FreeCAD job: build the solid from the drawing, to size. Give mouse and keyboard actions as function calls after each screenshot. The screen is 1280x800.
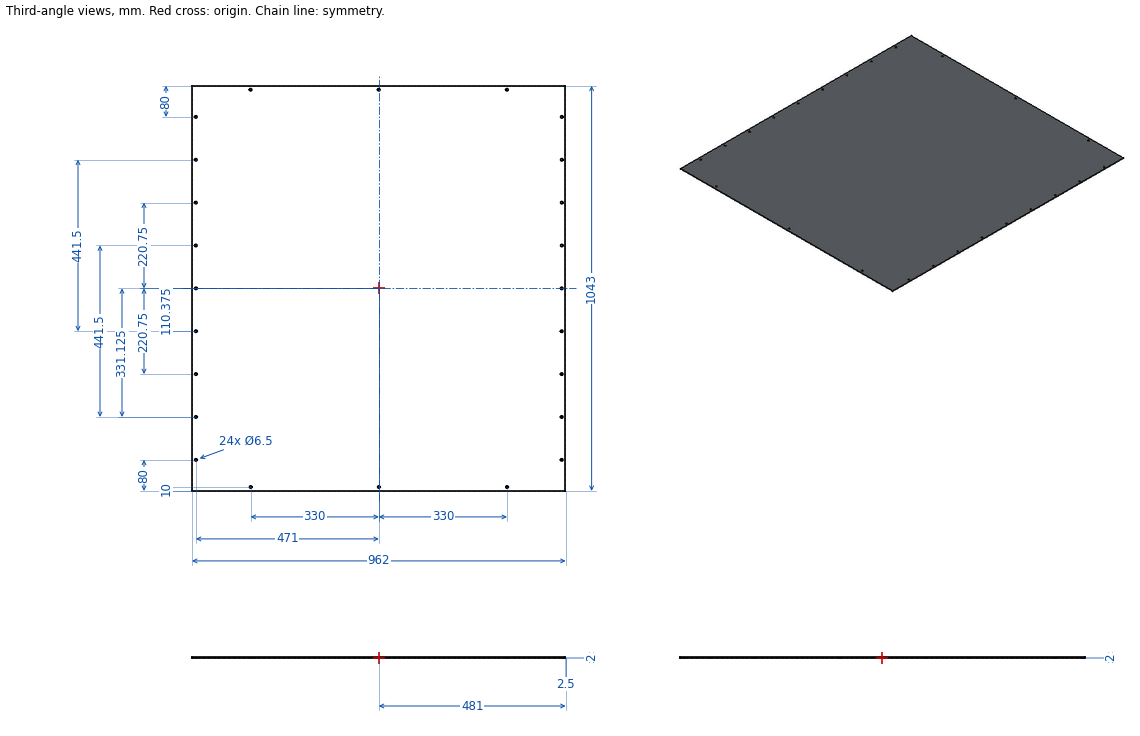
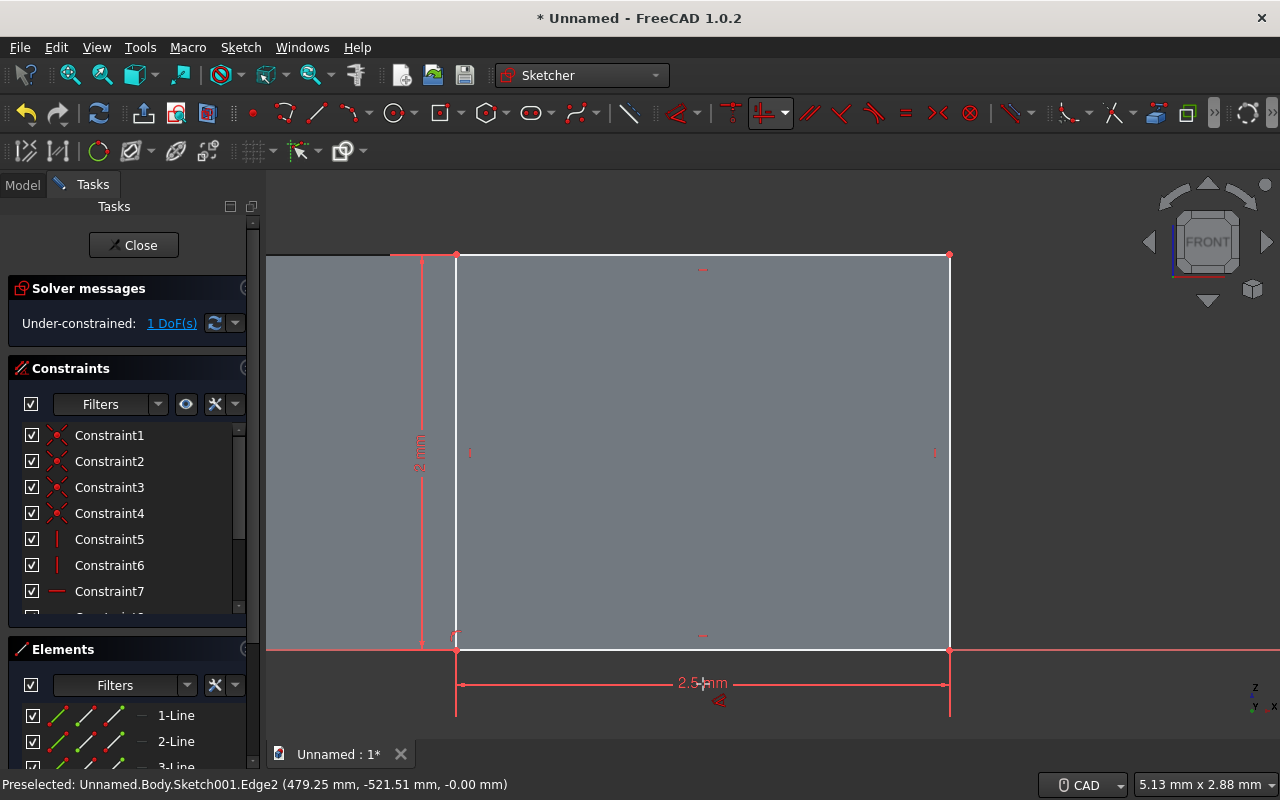
click(950, 650)
click(622, 684)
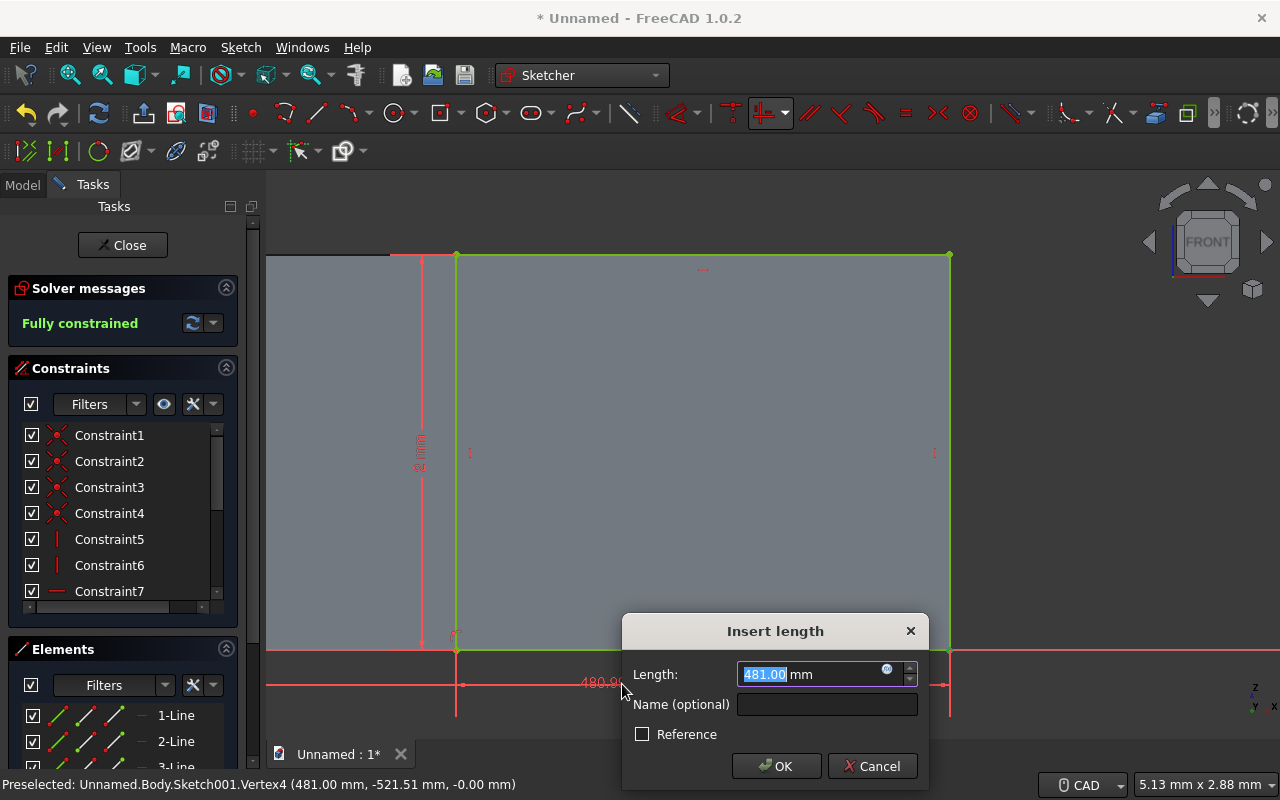
text(481)
key(Return)
key(Escape)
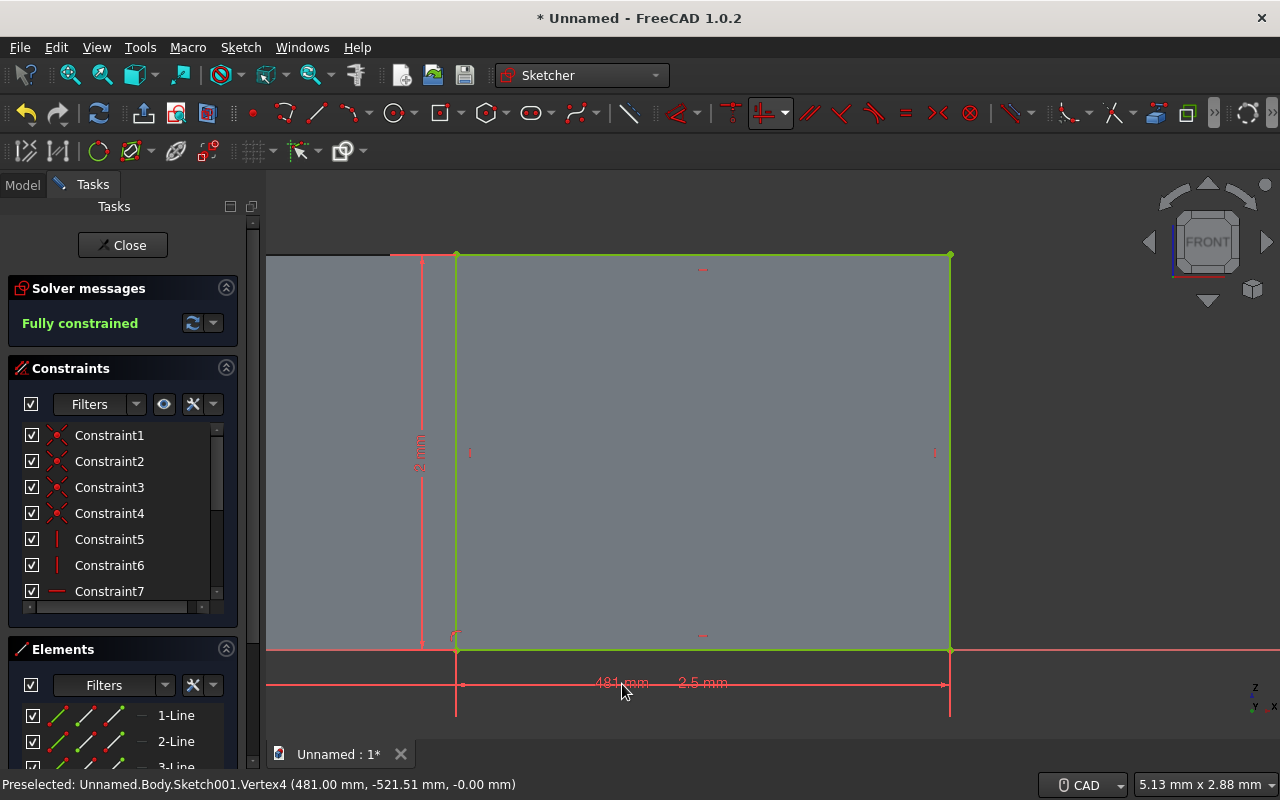
click(123, 245)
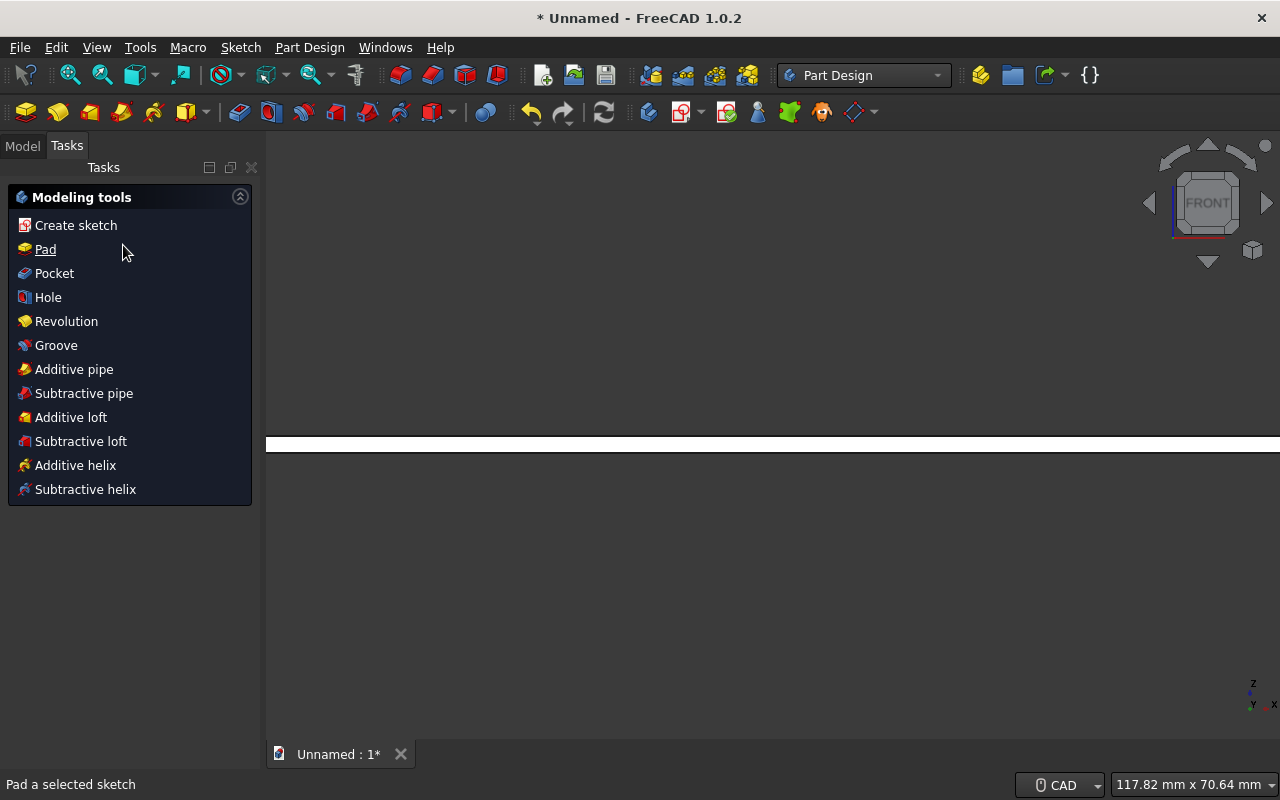
click(240, 112)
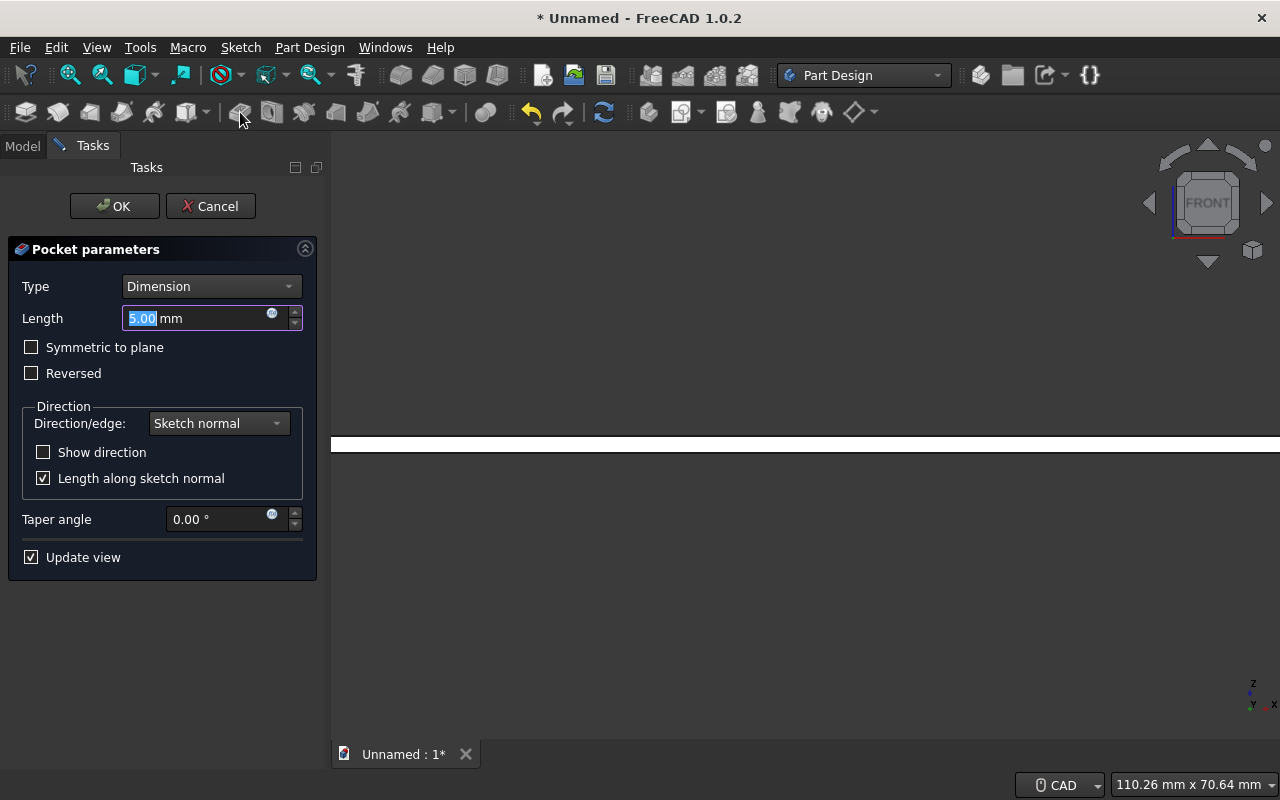
click(212, 286)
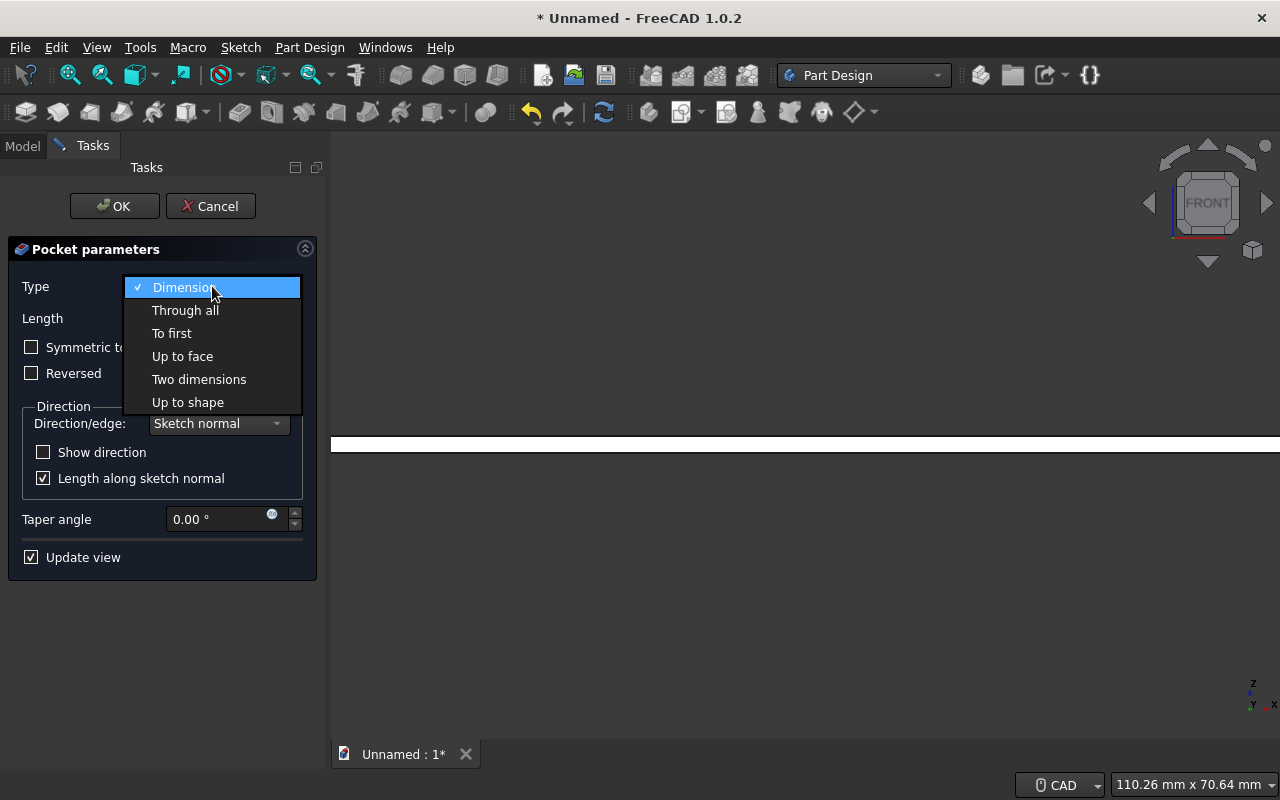
click(212, 310)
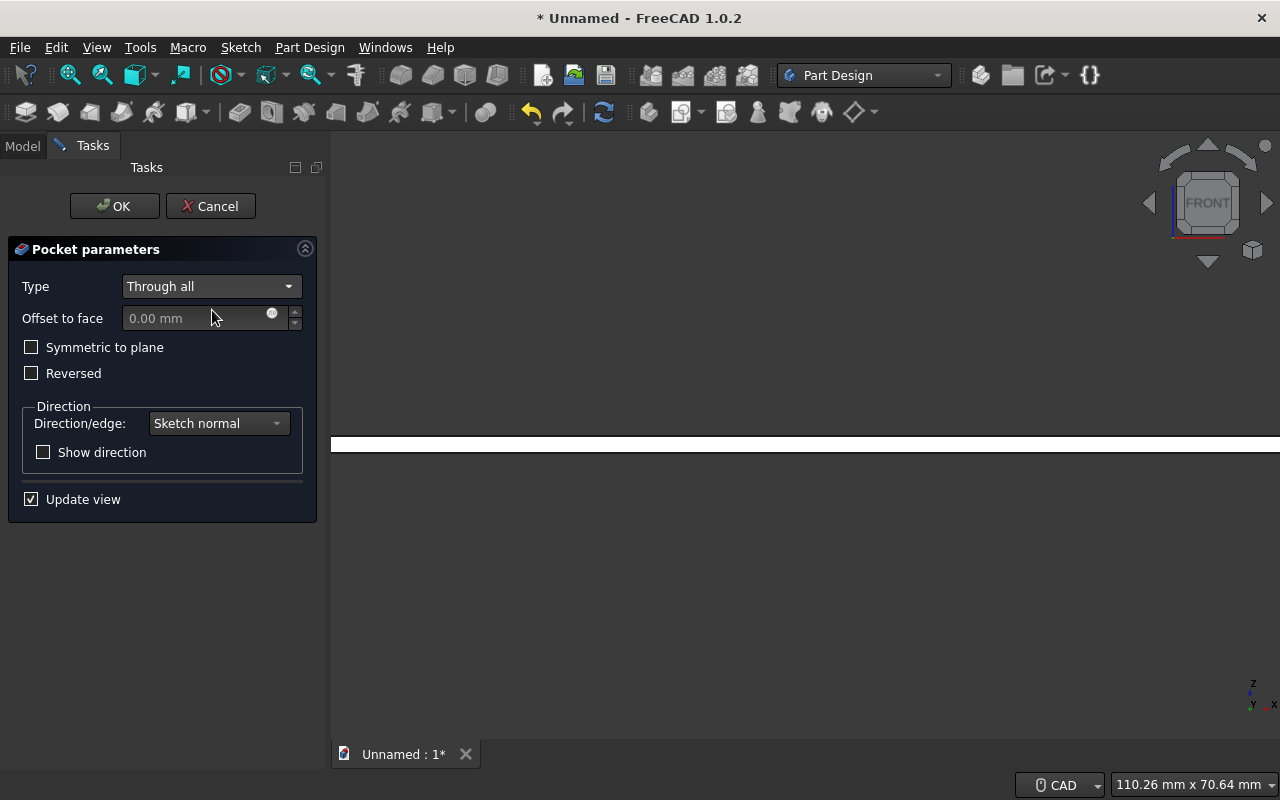
click(115, 206)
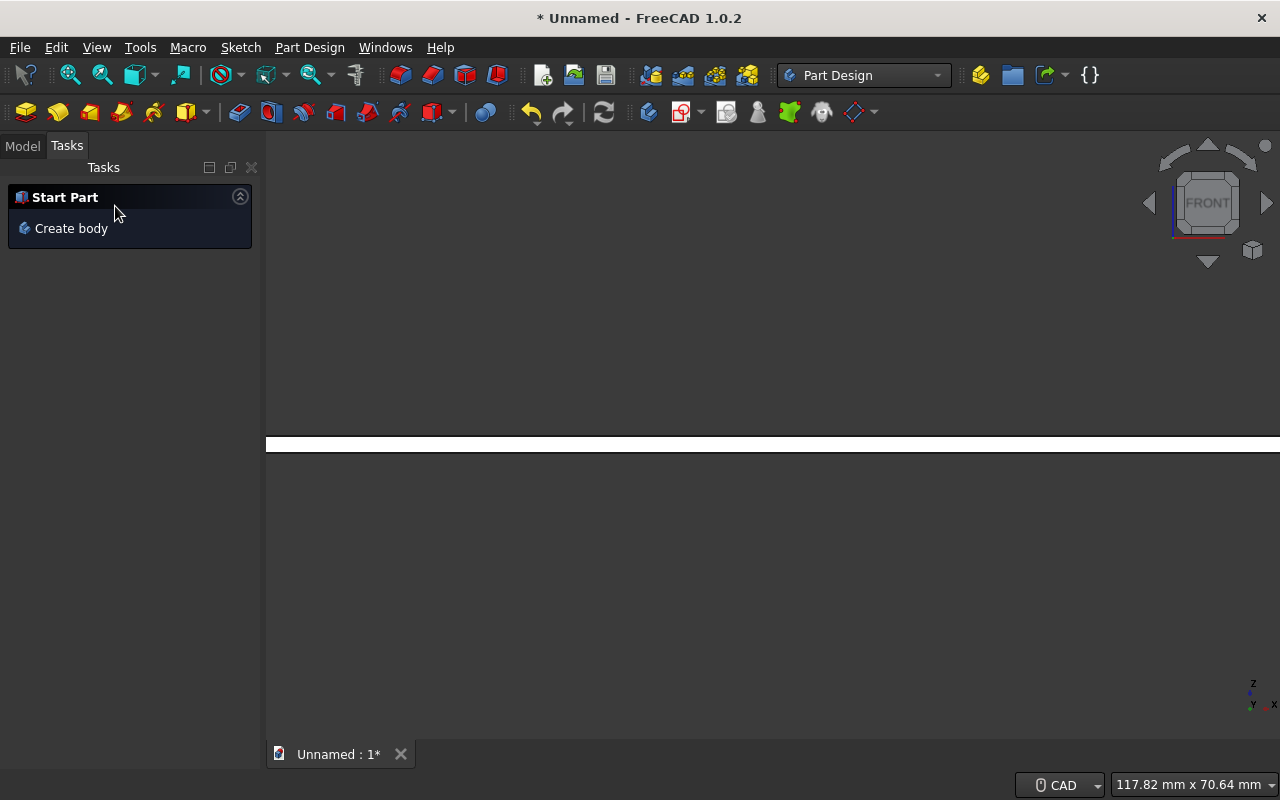
key(0)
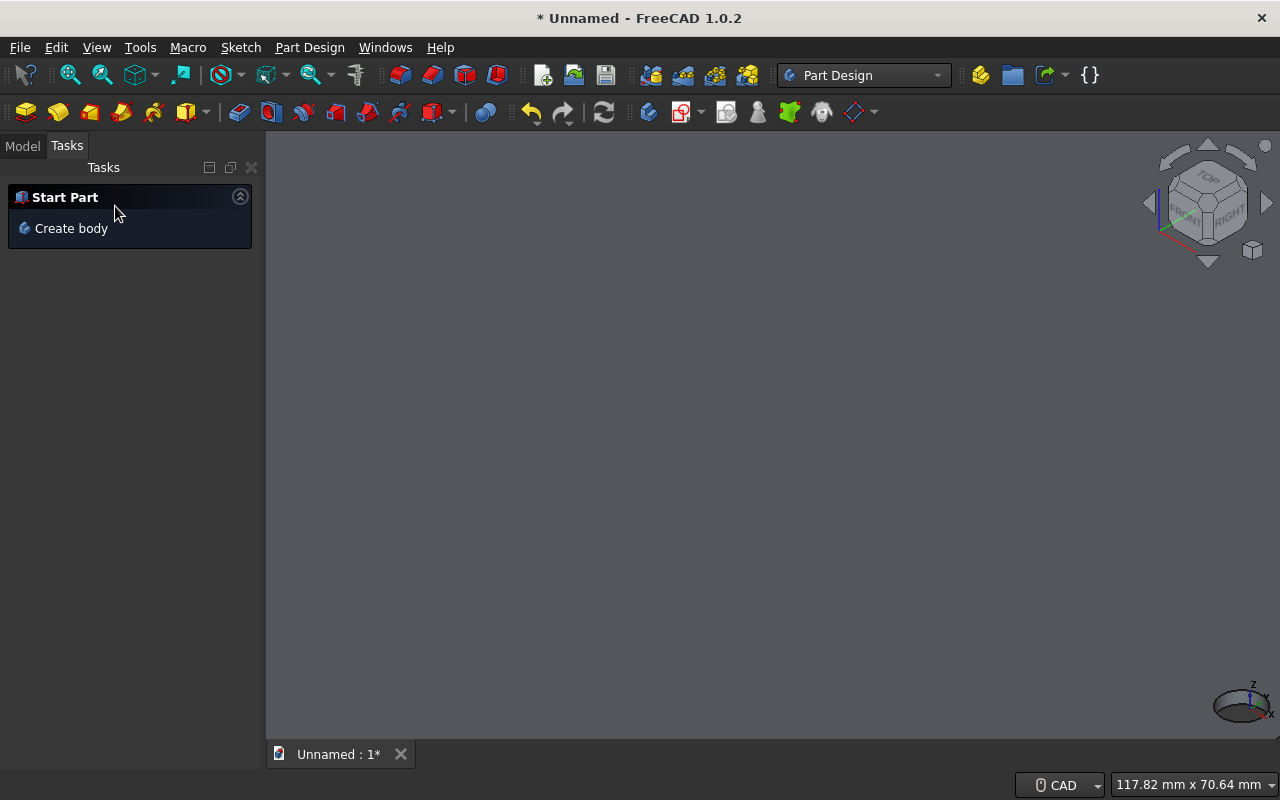
key(v)
key(f)